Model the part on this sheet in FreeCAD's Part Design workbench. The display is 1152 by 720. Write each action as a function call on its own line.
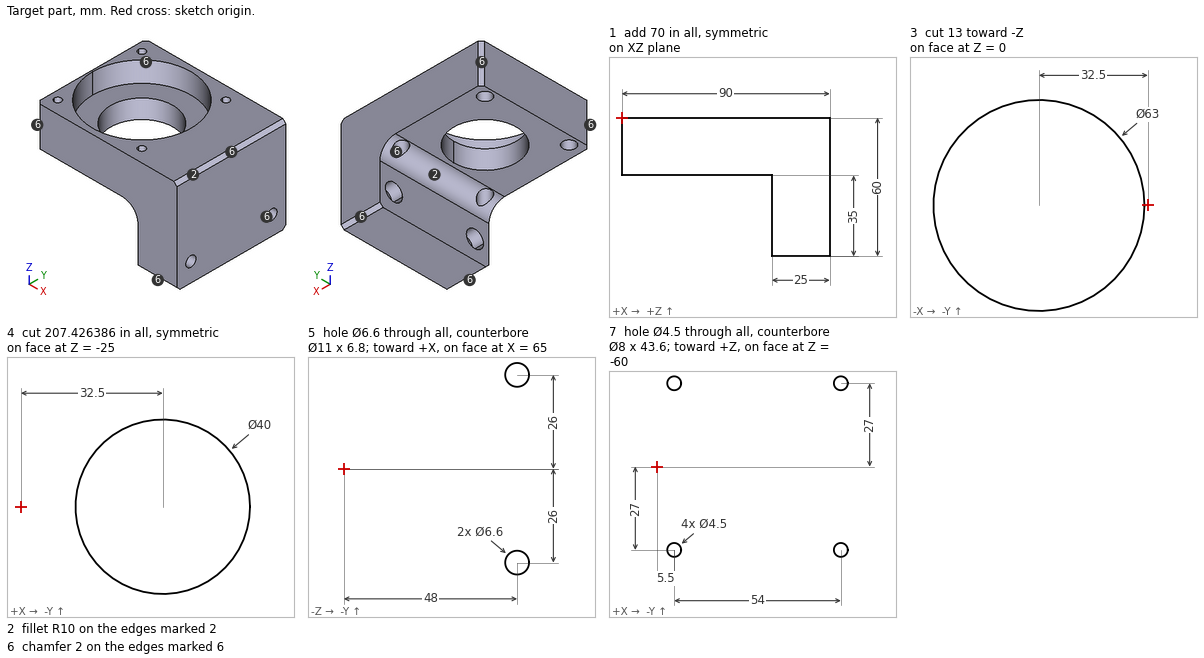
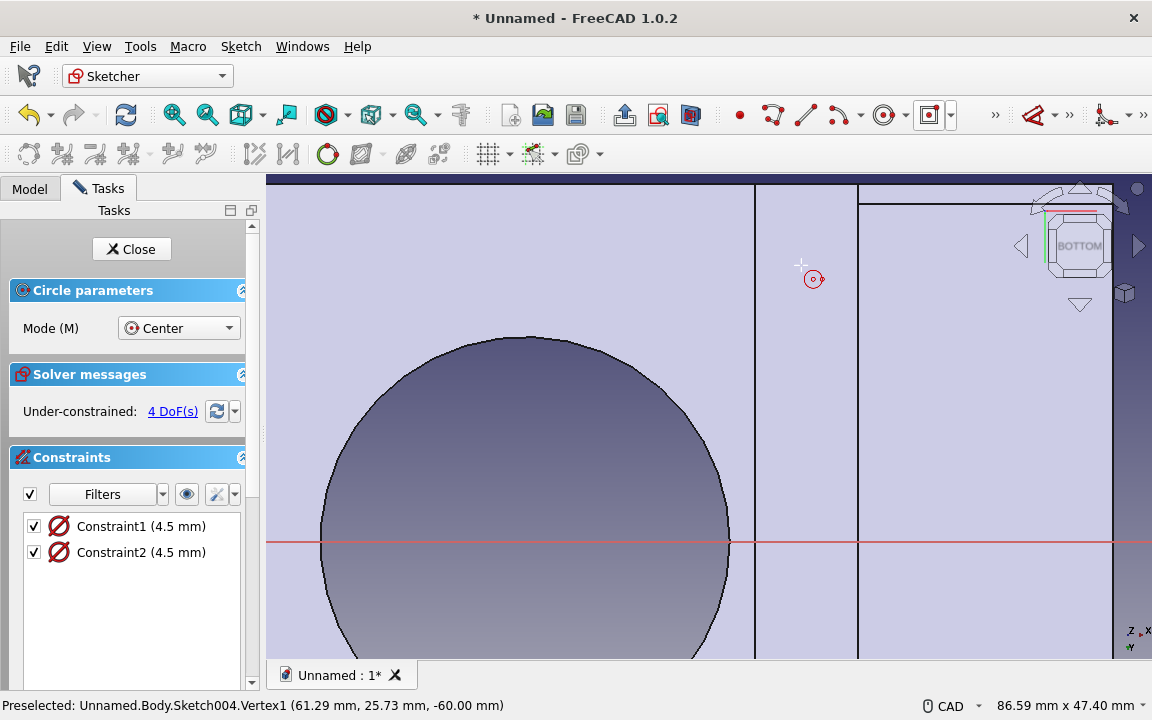
click(801, 265)
move(818, 249)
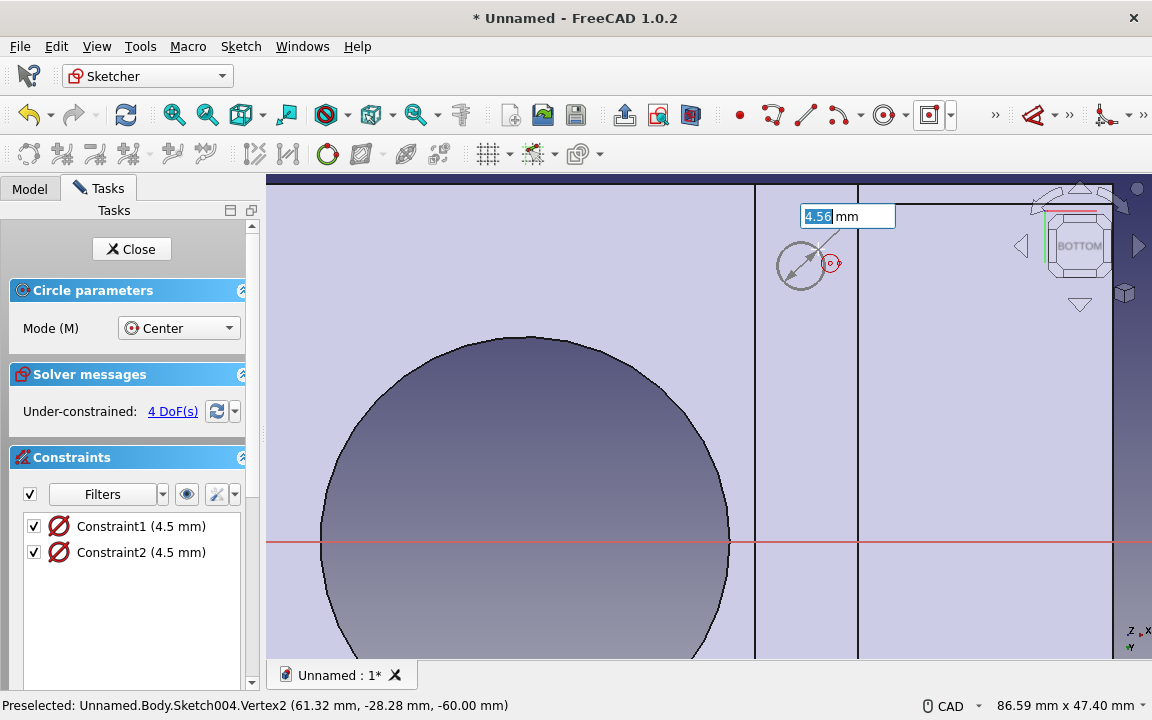
text(4.5)
key(Return)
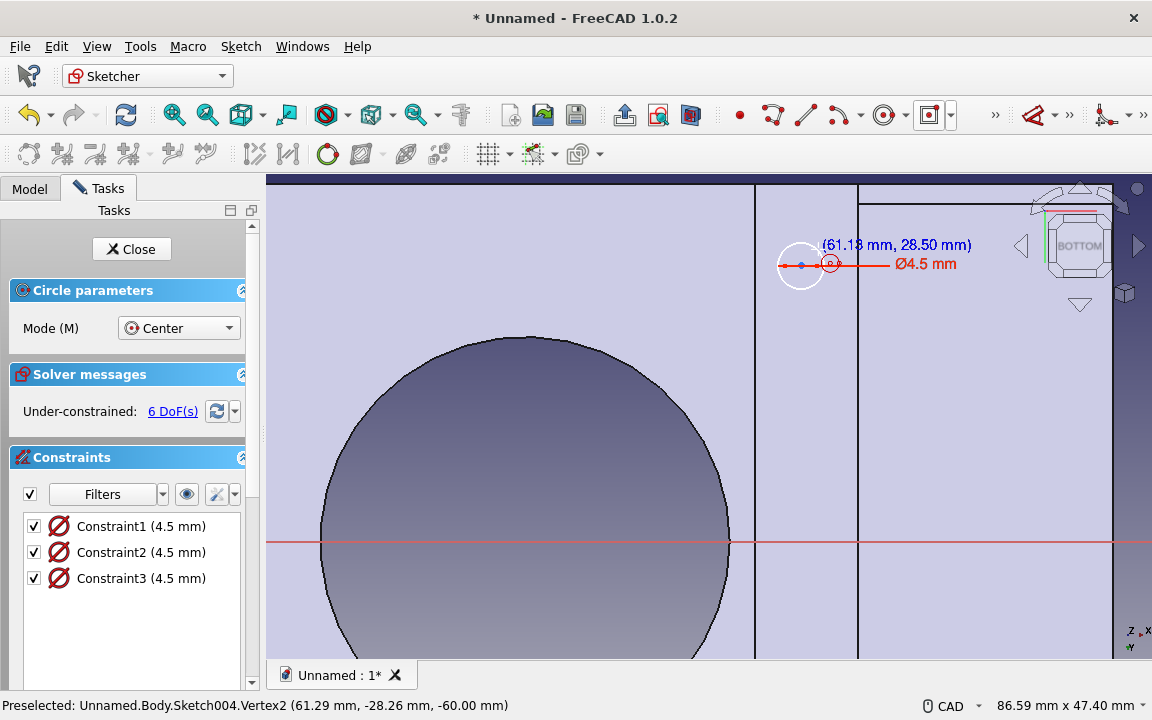
scroll(801, 264, down, 3)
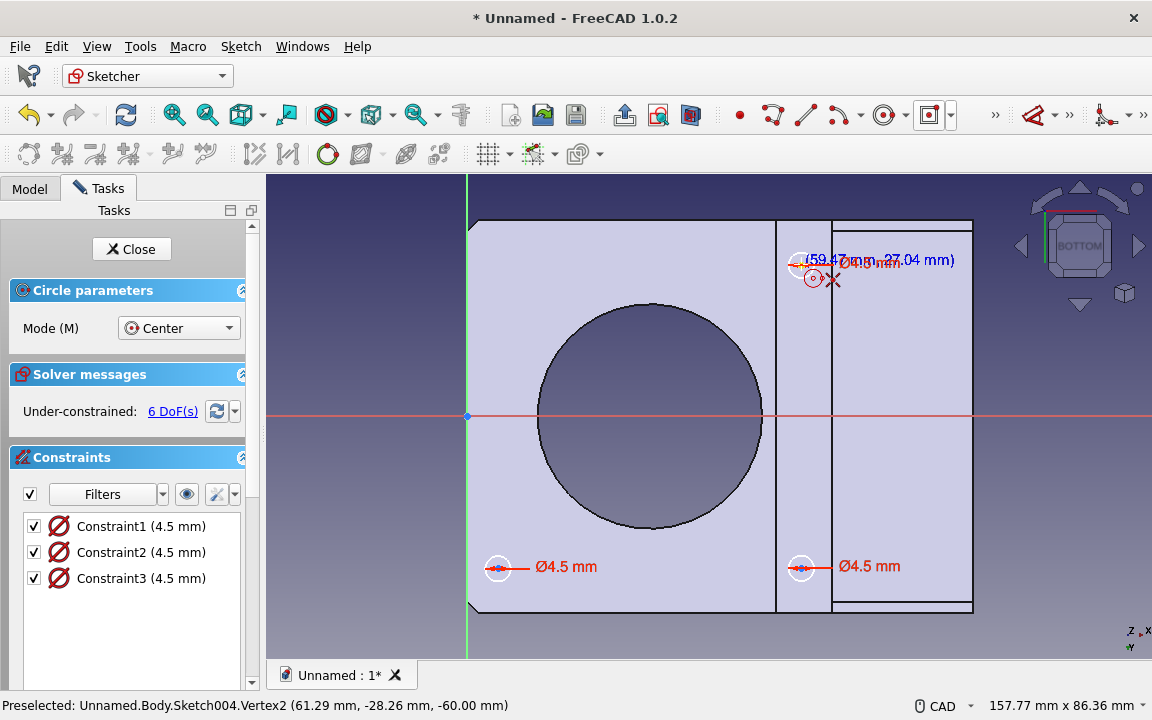
scroll(498, 265, up, 3)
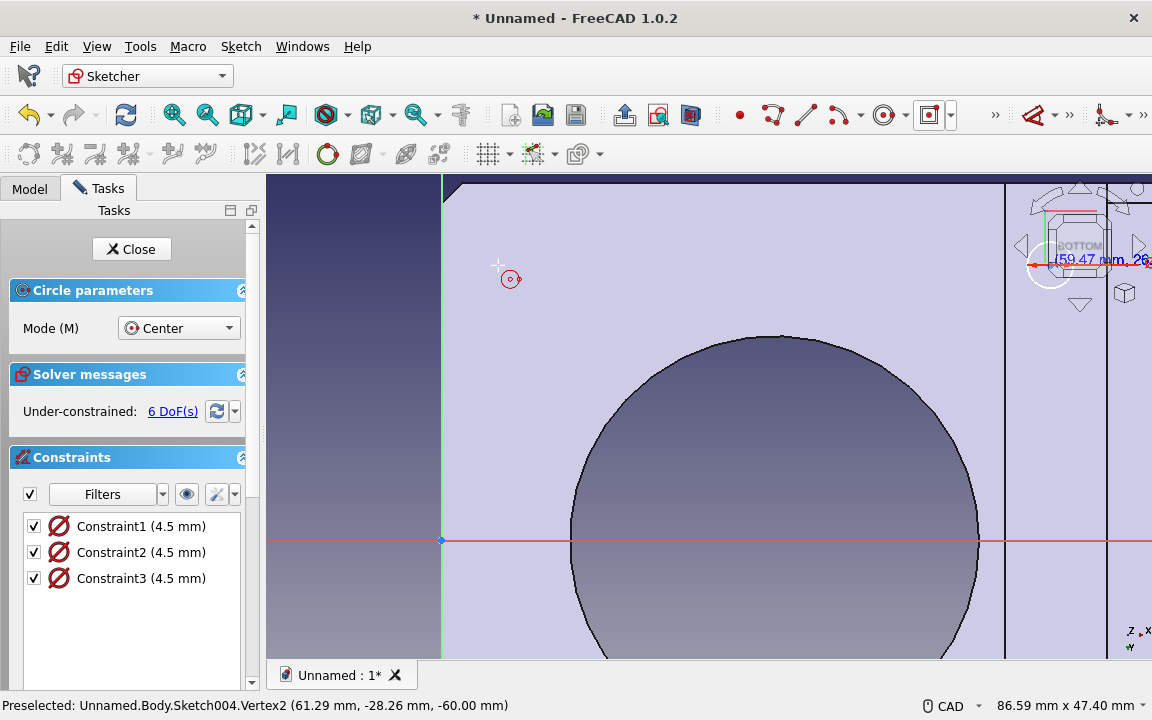
click(498, 265)
move(514, 248)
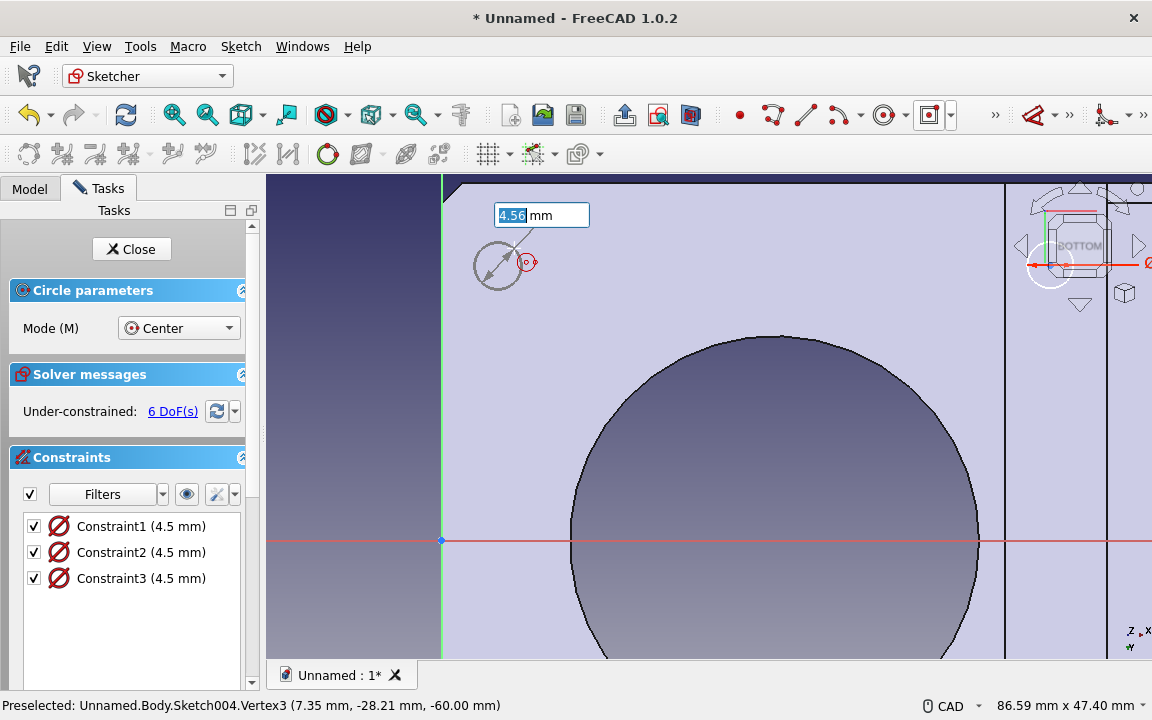
text(4.5)
key(Return)
key(Escape)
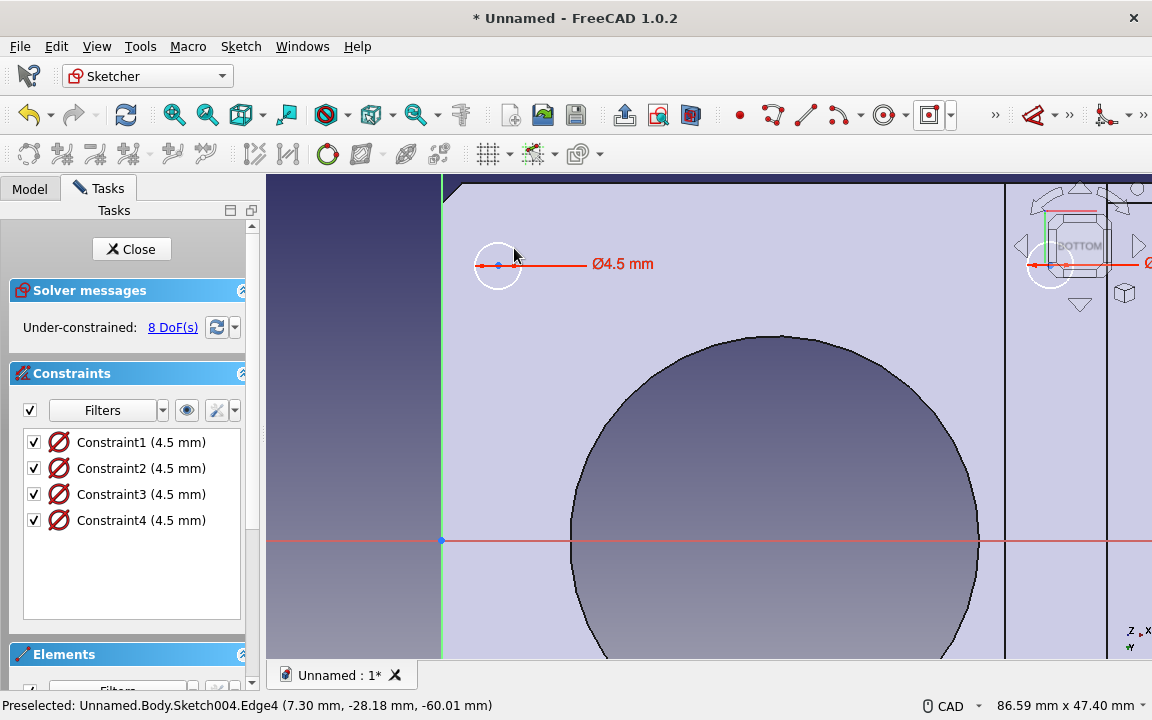
scroll(498, 265, down, 3)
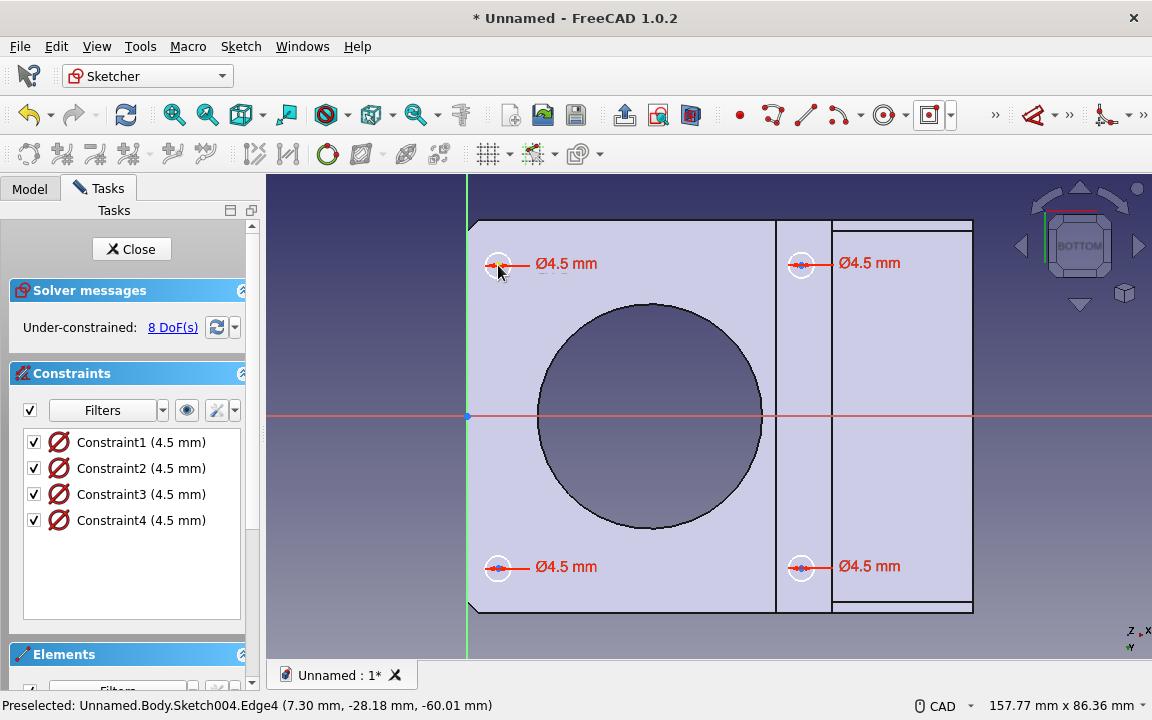
click(498, 569)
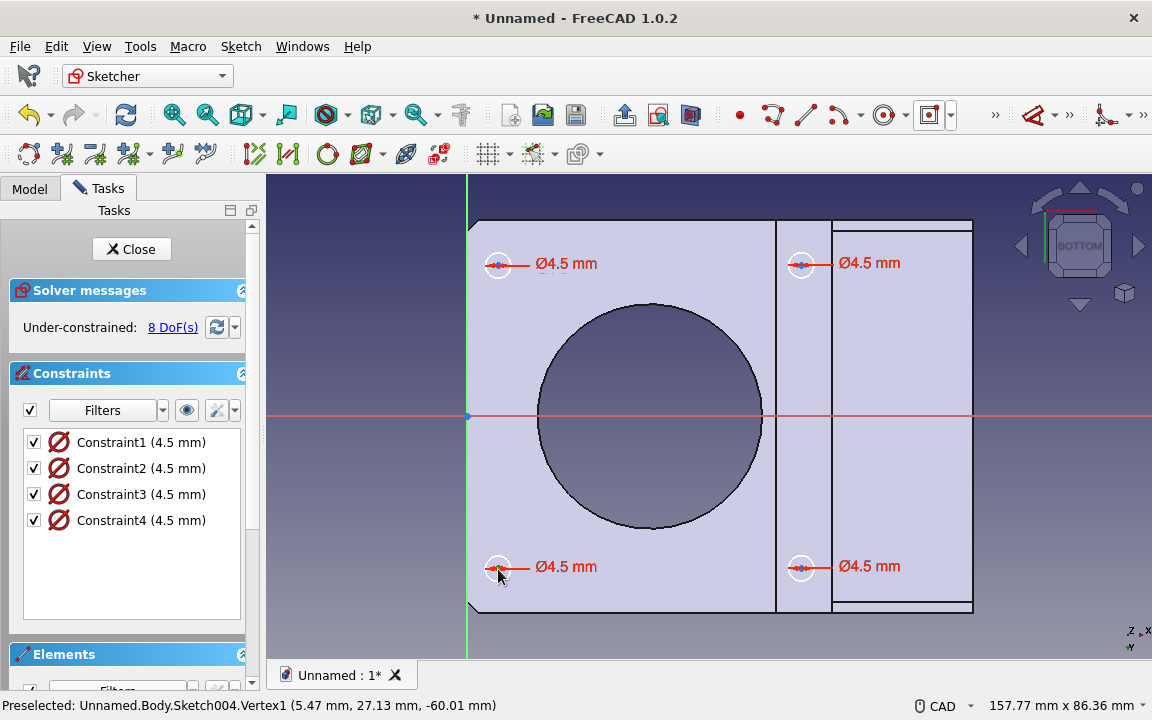
click(801, 568)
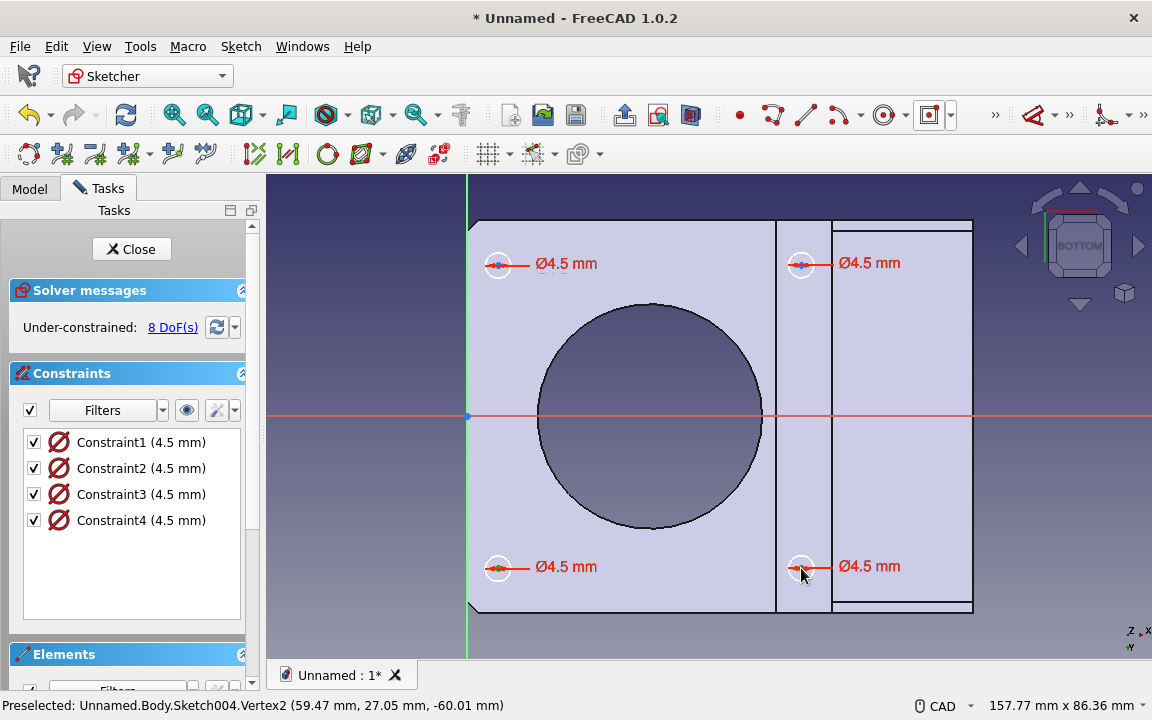
key(h)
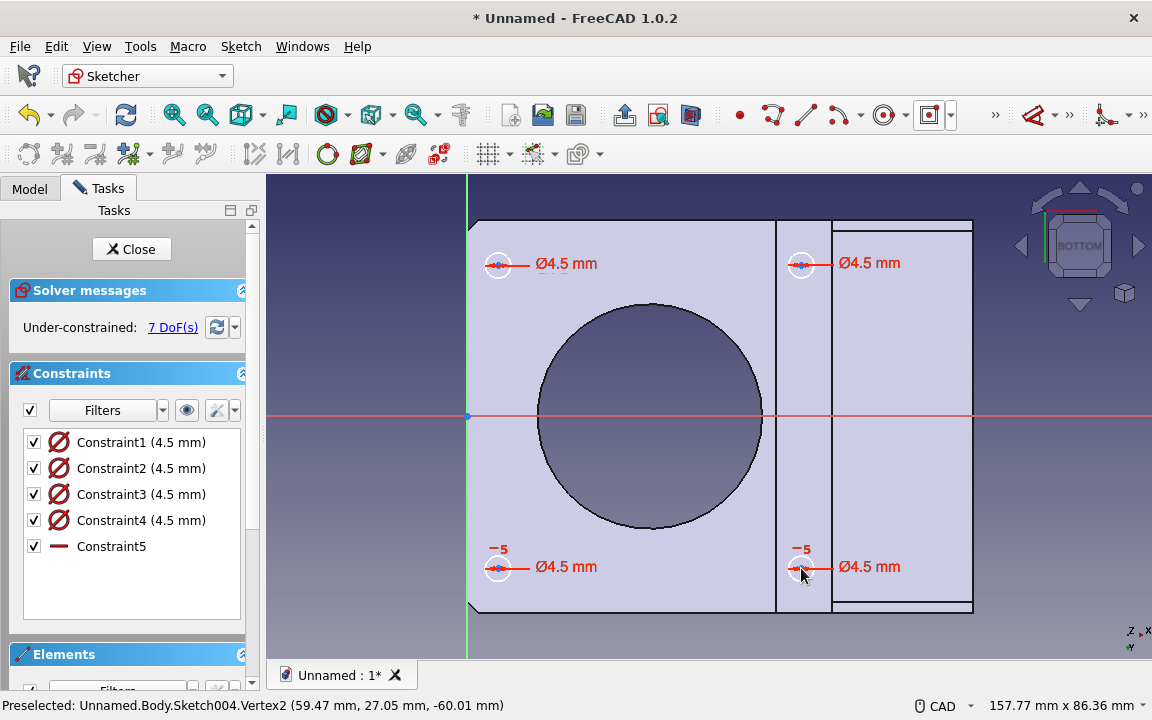
click(801, 569)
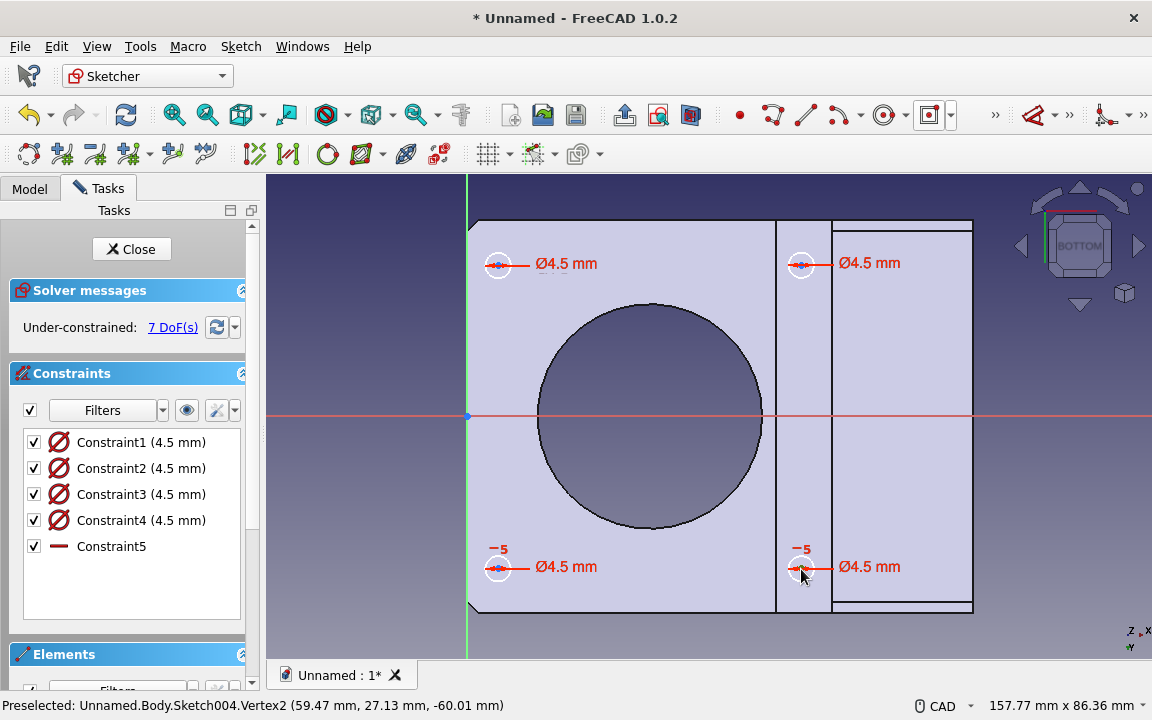
click(801, 265)